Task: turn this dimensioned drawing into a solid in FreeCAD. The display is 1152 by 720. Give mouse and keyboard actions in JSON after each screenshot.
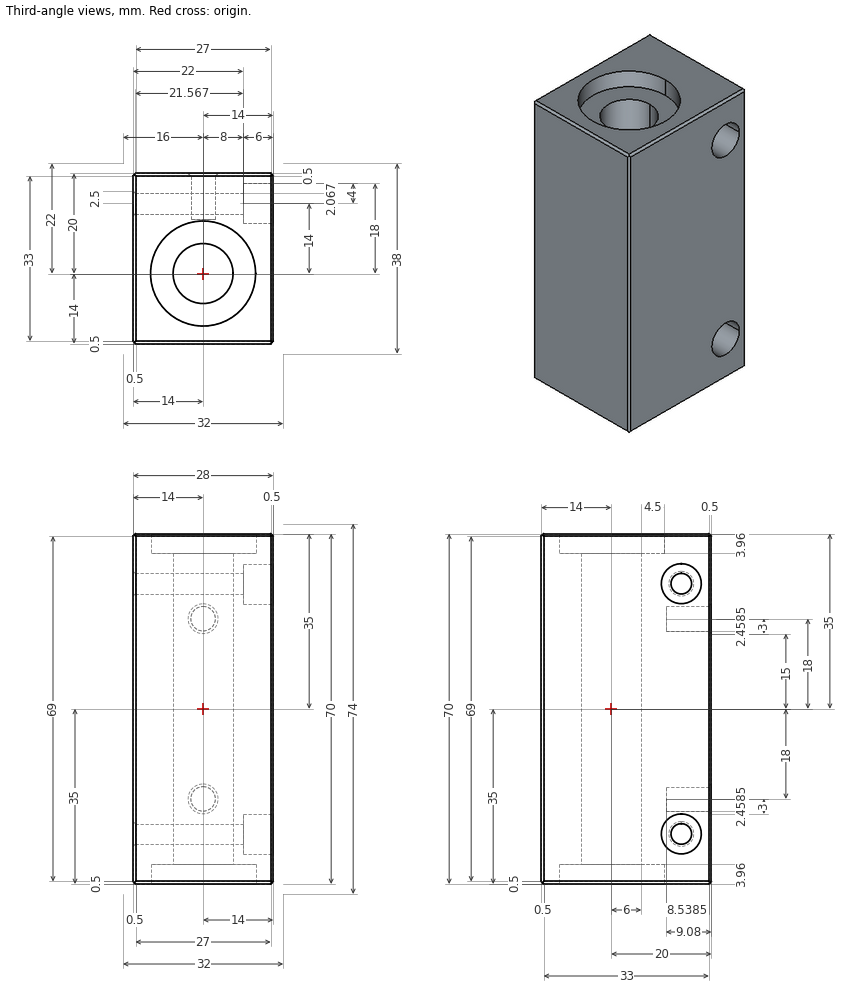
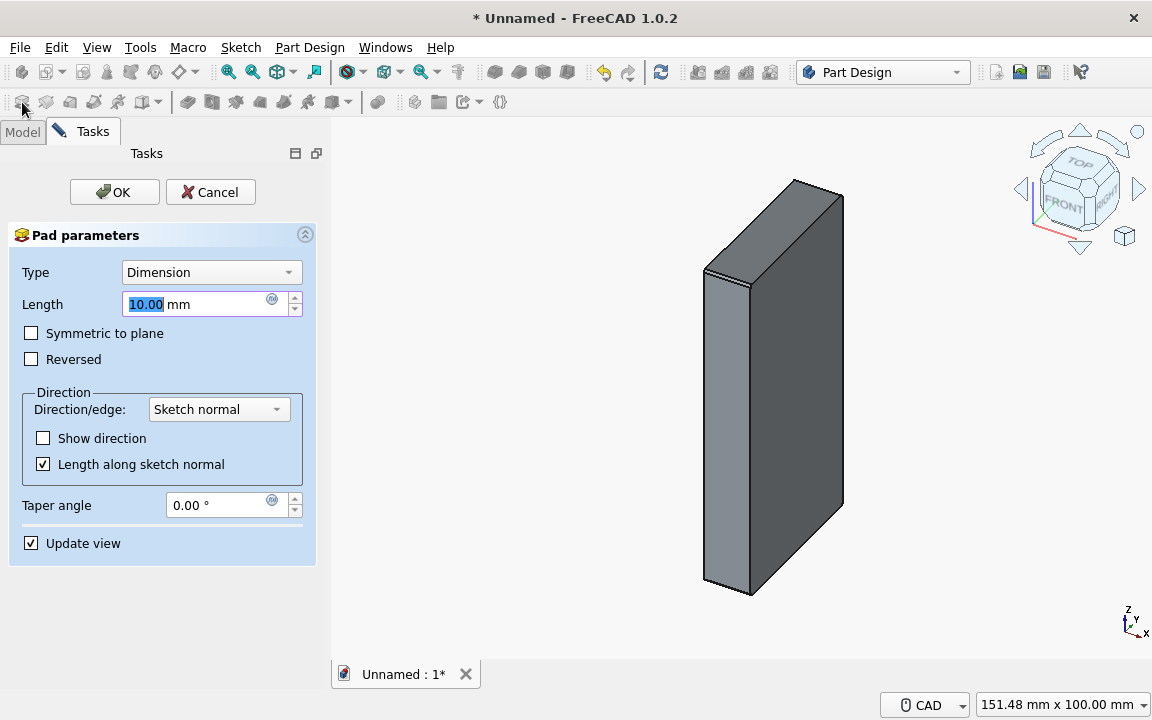
{"action": "type", "text": "28"}
{"action": "key", "text": "Tab"}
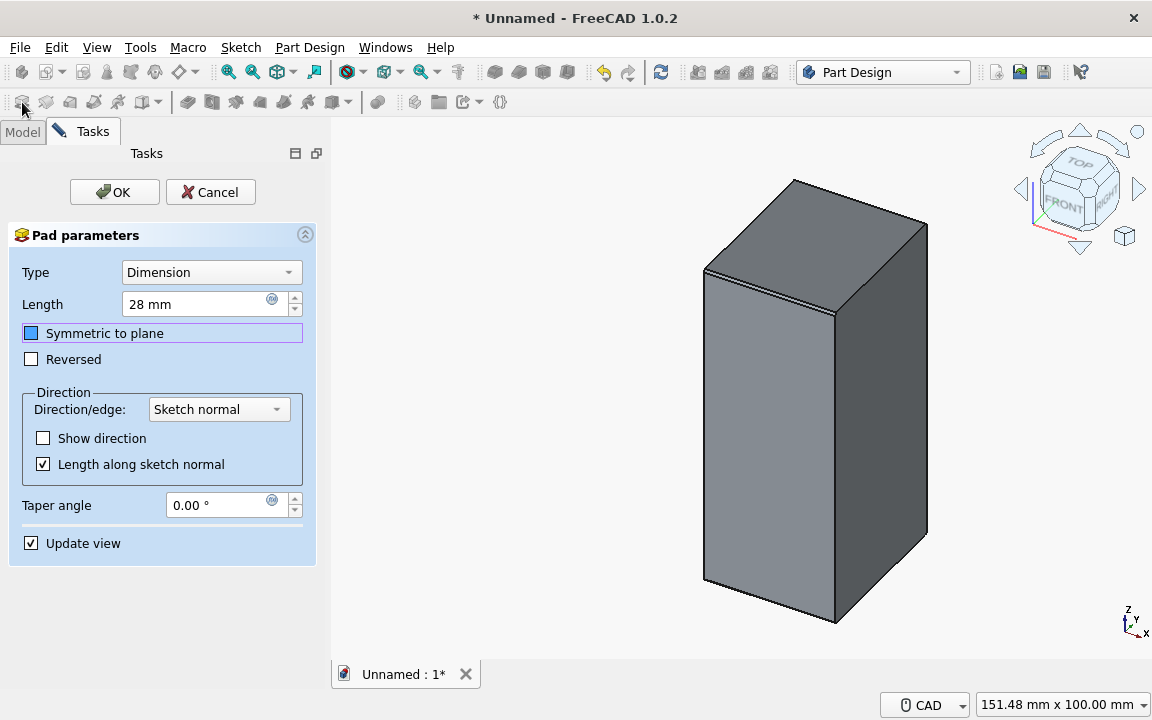
{"action": "left_click", "coordinate": [30, 333]}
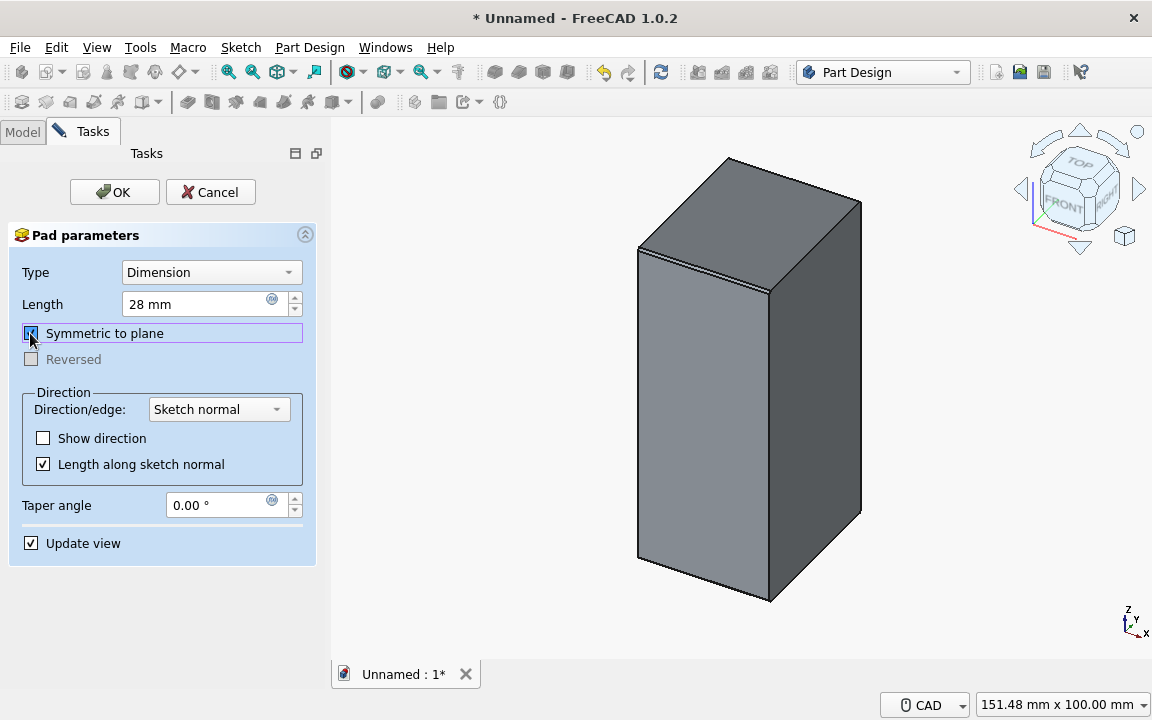
{"action": "left_click", "coordinate": [115, 192]}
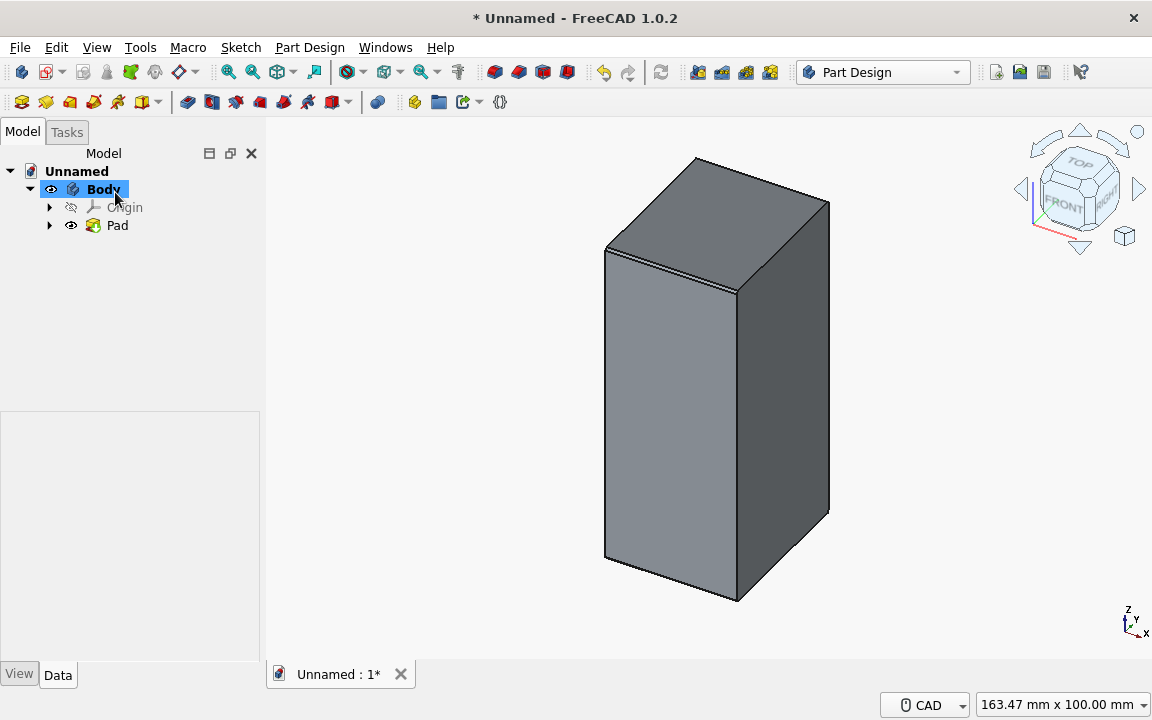
{"action": "left_click", "coordinate": [46, 72]}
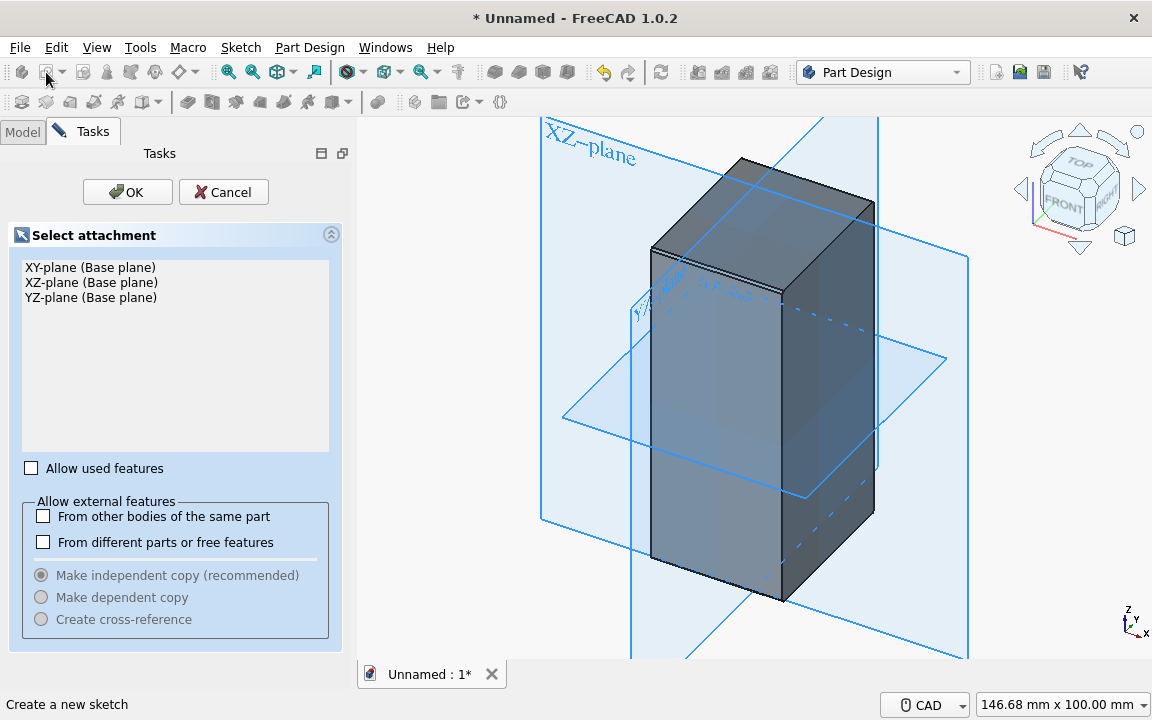
{"action": "left_click", "coordinate": [82, 298]}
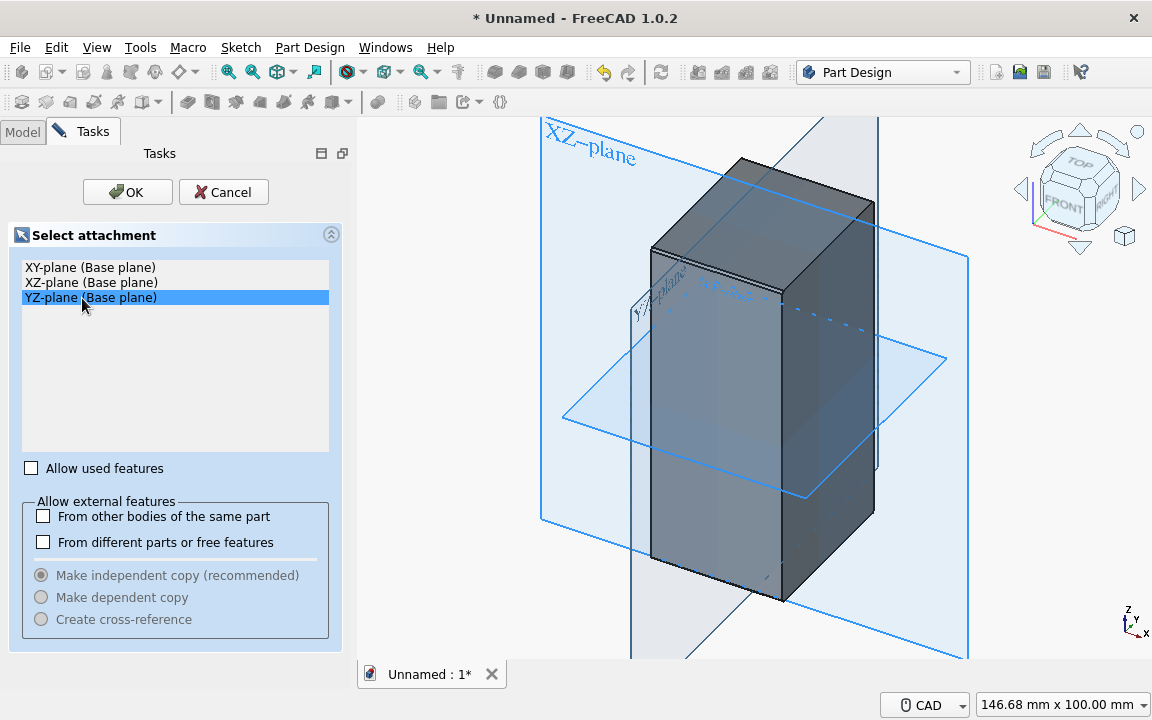
{"action": "left_click", "coordinate": [128, 192]}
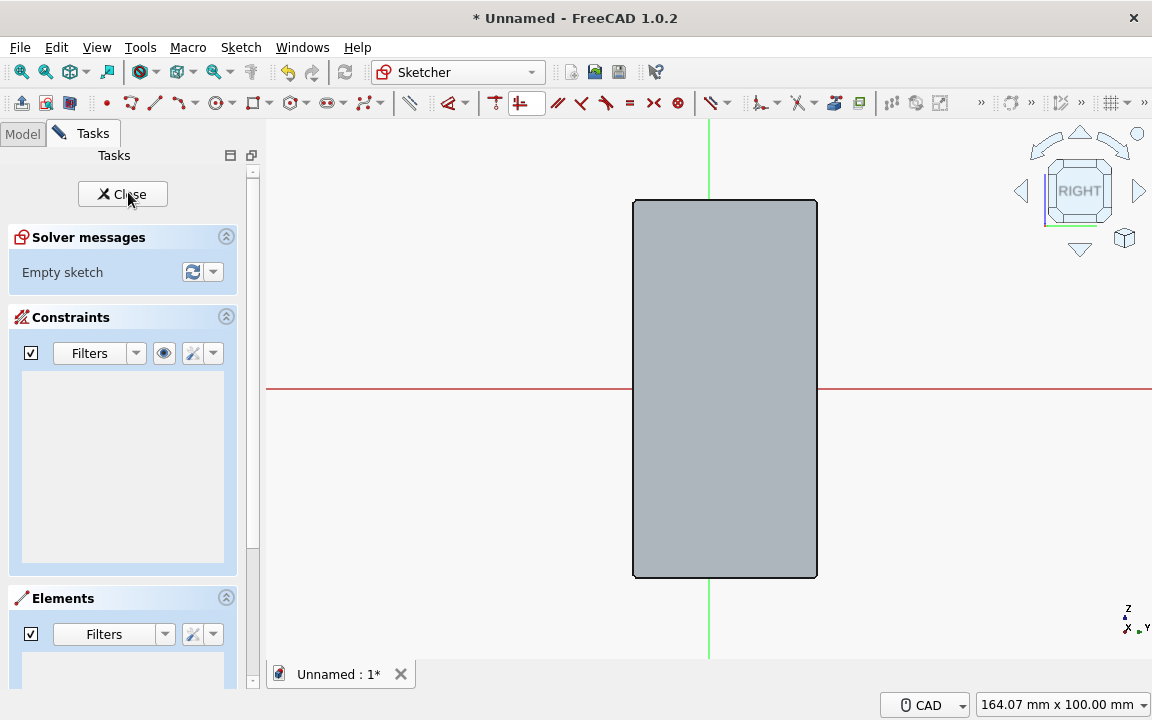
{"action": "key", "text": "q s"}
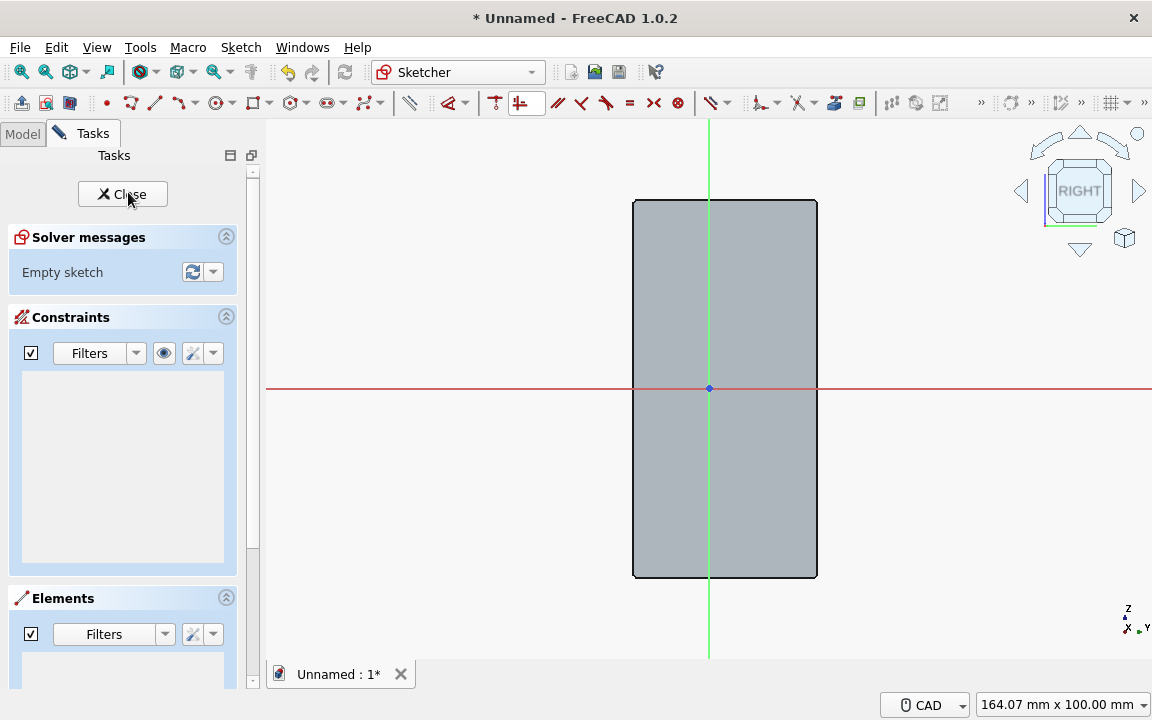
{"action": "left_click", "coordinate": [132, 104]}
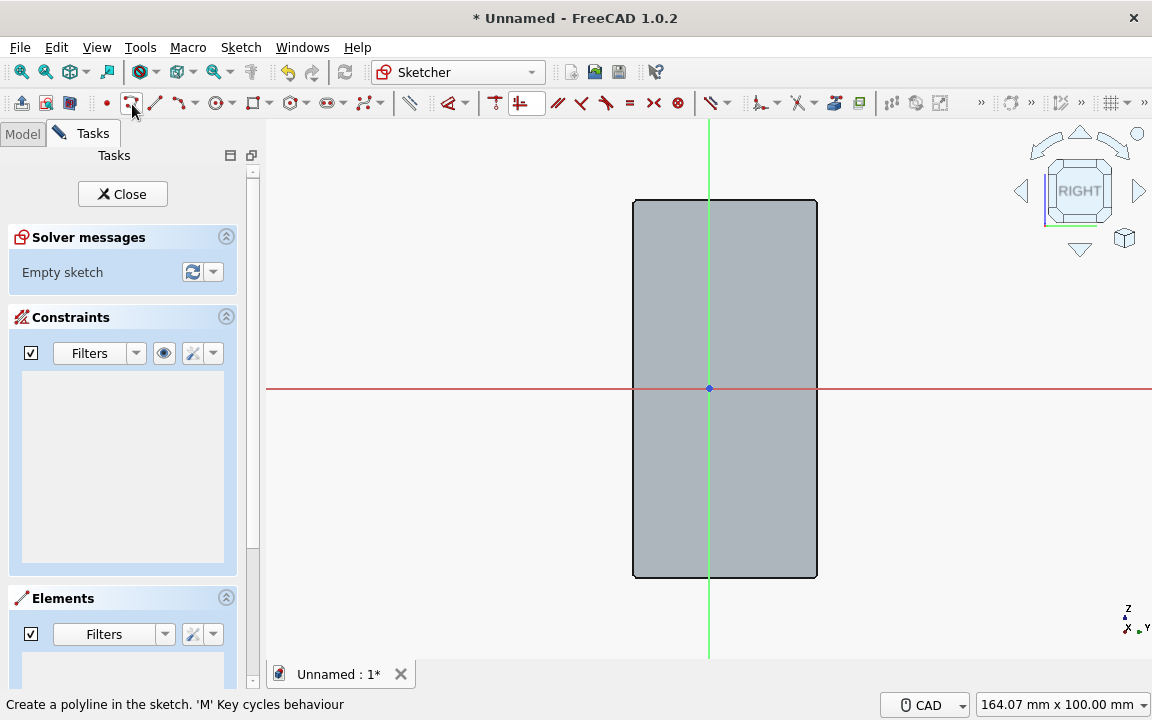
{"action": "left_click", "coordinate": [741, 557]}
{"action": "left_click", "coordinate": [741, 221]}
{"action": "left_click", "coordinate": [766, 221]}
{"action": "left_click", "coordinate": [766, 200]}
{"action": "left_click", "coordinate": [709, 200]}
{"action": "left_click", "coordinate": [718, 578]}
{"action": "left_click", "coordinate": [766, 578]}
{"action": "left_click", "coordinate": [766, 557]}
{"action": "left_click", "coordinate": [741, 558]}
{"action": "key", "text": "Escape"}
{"action": "key", "text": "Escape"}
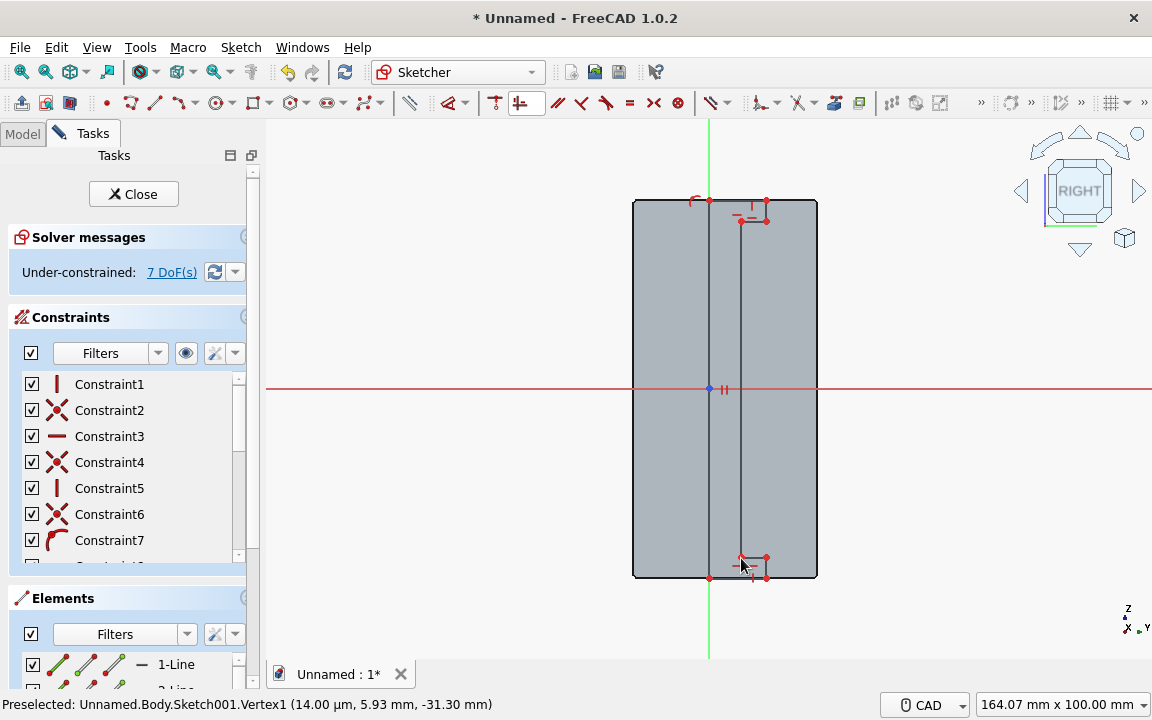
{"action": "key", "text": "d"}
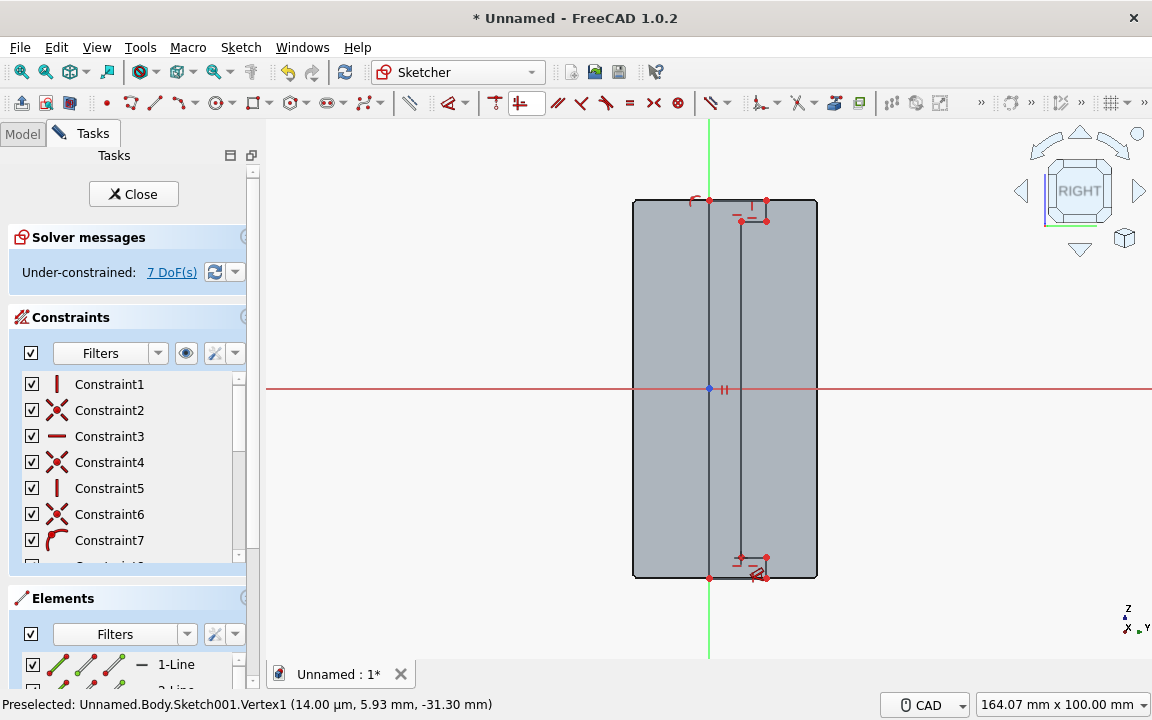
{"action": "left_click", "coordinate": [709, 314]}
{"action": "left_click", "coordinate": [675, 303]}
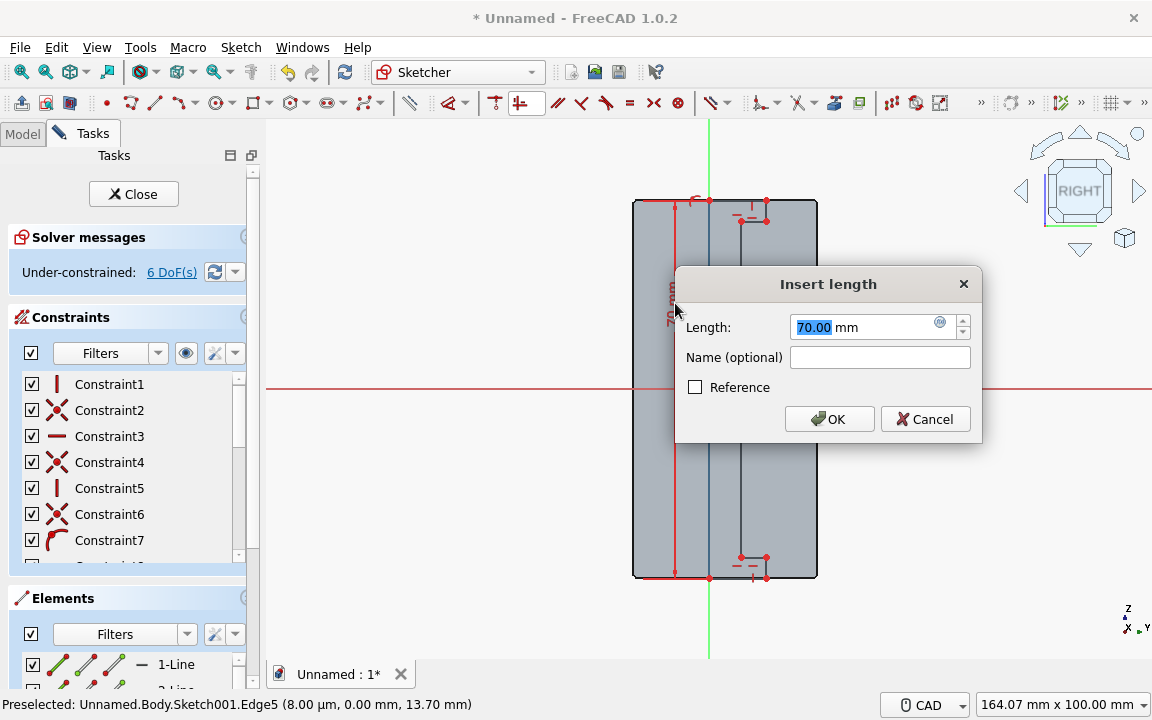
{"action": "type", "text": "70"}
{"action": "key", "text": "Return"}